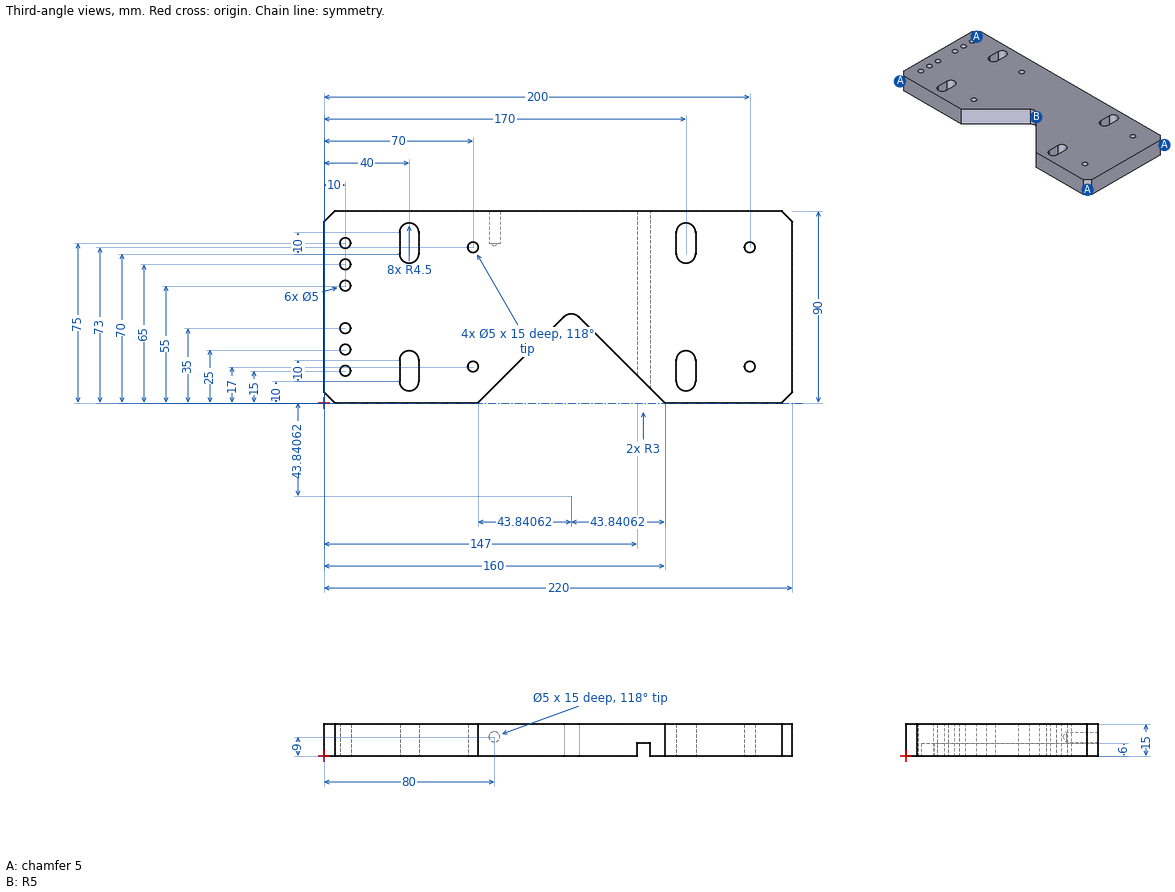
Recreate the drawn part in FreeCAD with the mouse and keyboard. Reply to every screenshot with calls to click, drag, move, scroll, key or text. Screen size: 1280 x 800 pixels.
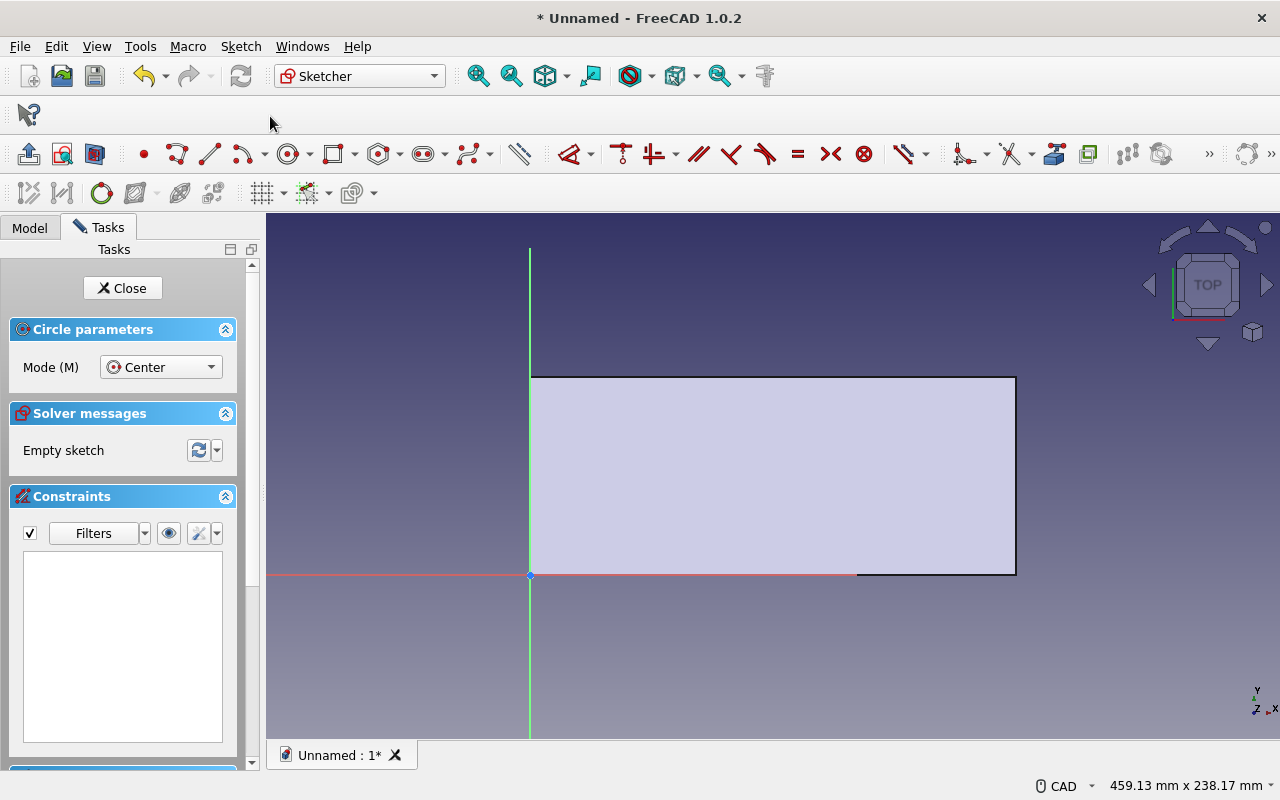
scroll(685, 414, up, 8)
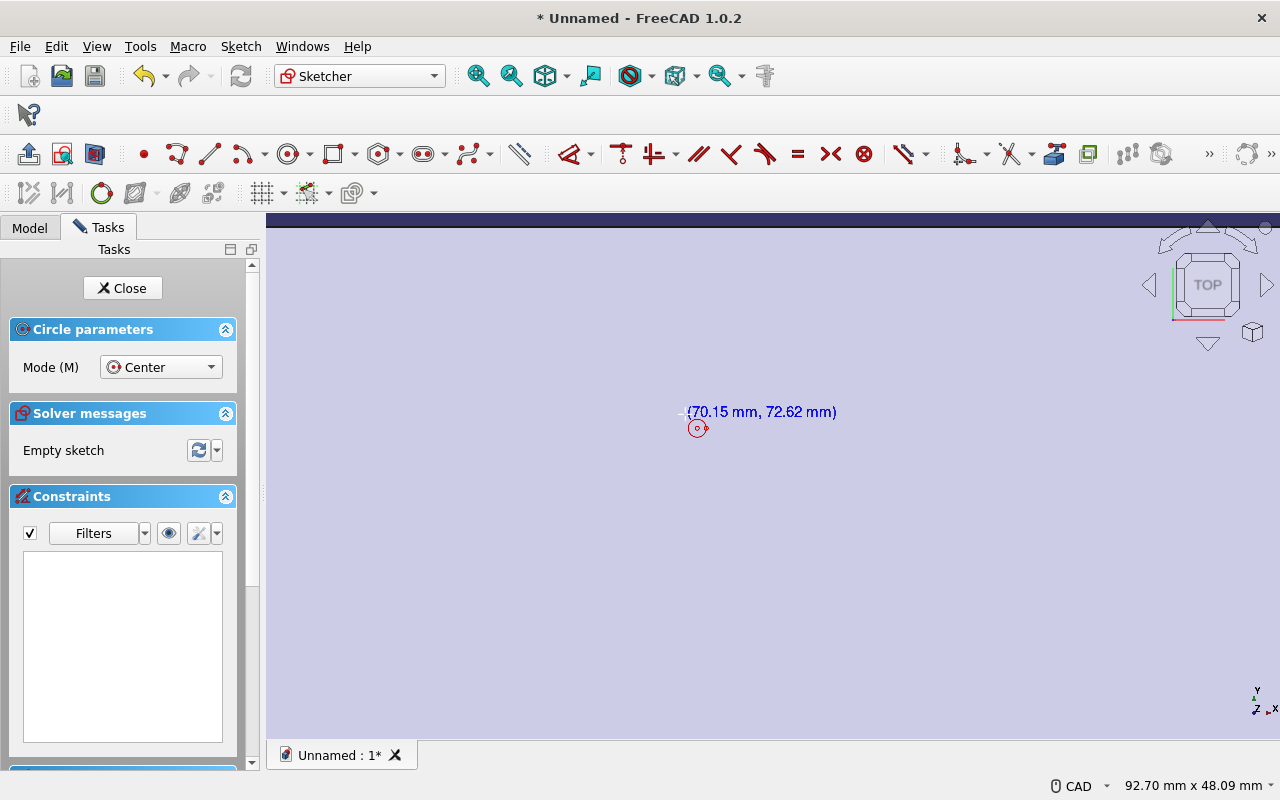
scroll(600, 370, down, 7)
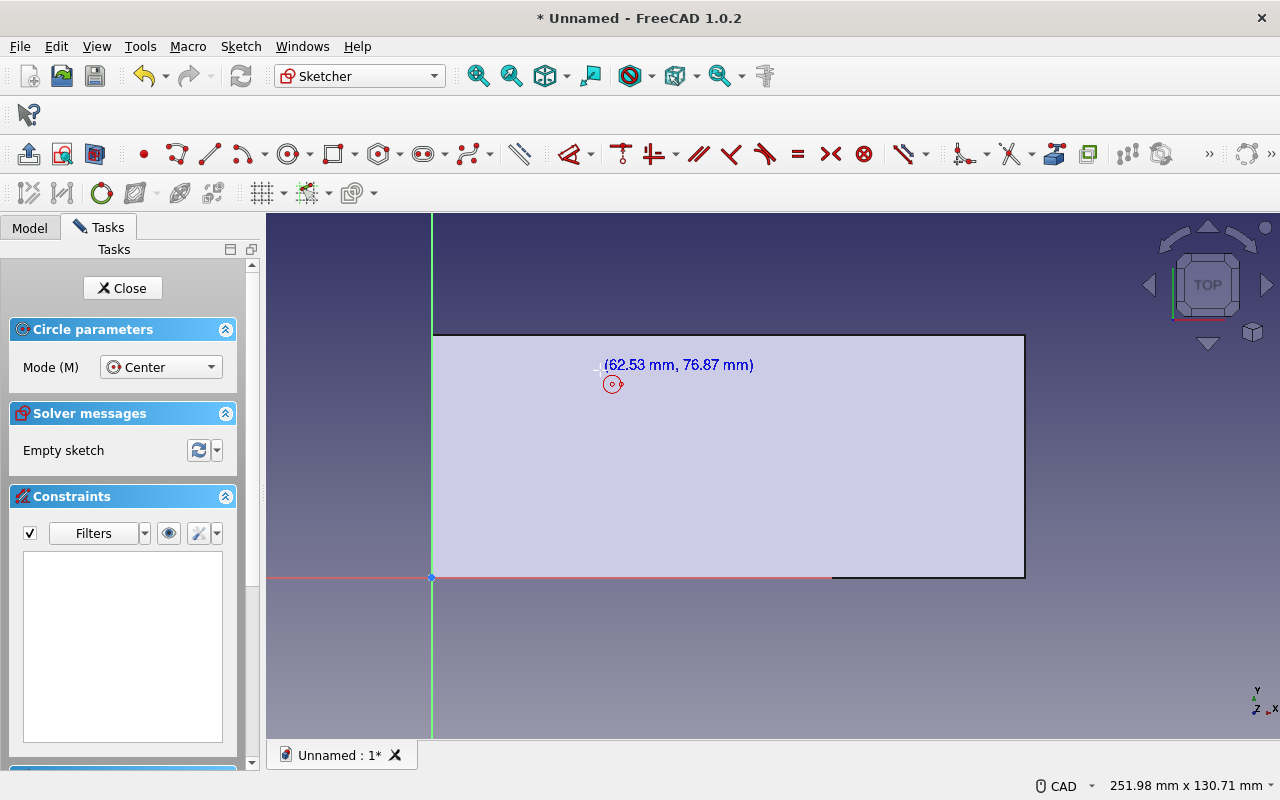
click(620, 381)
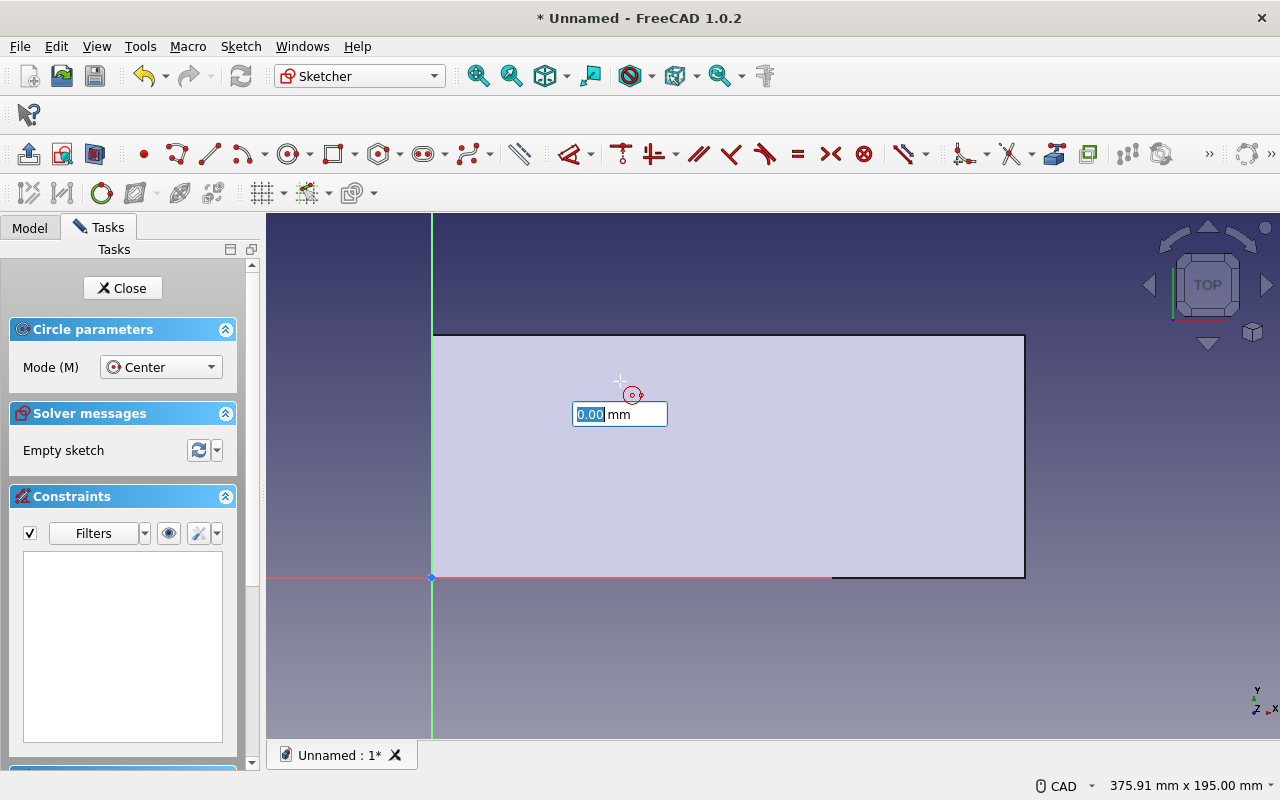
scroll(625, 376, up, 5)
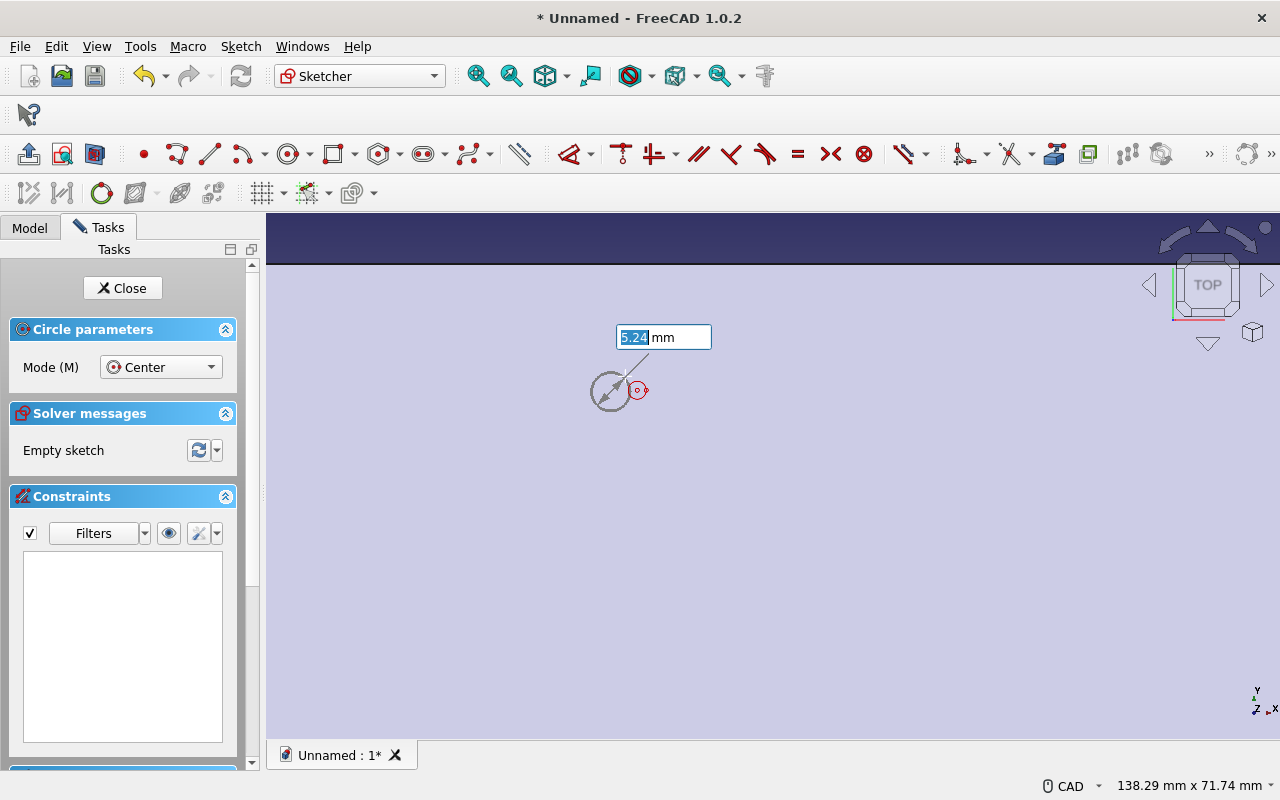
click(625, 376)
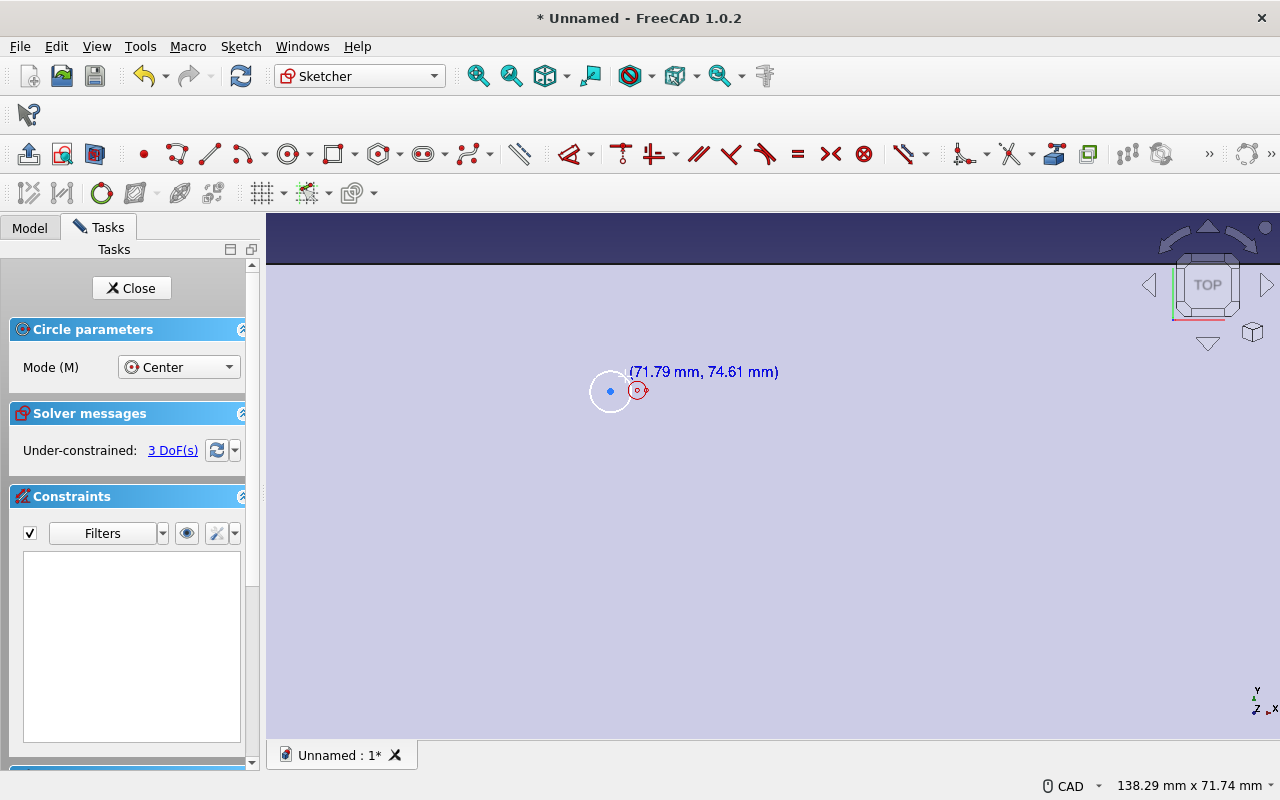
scroll(625, 376, down, 5)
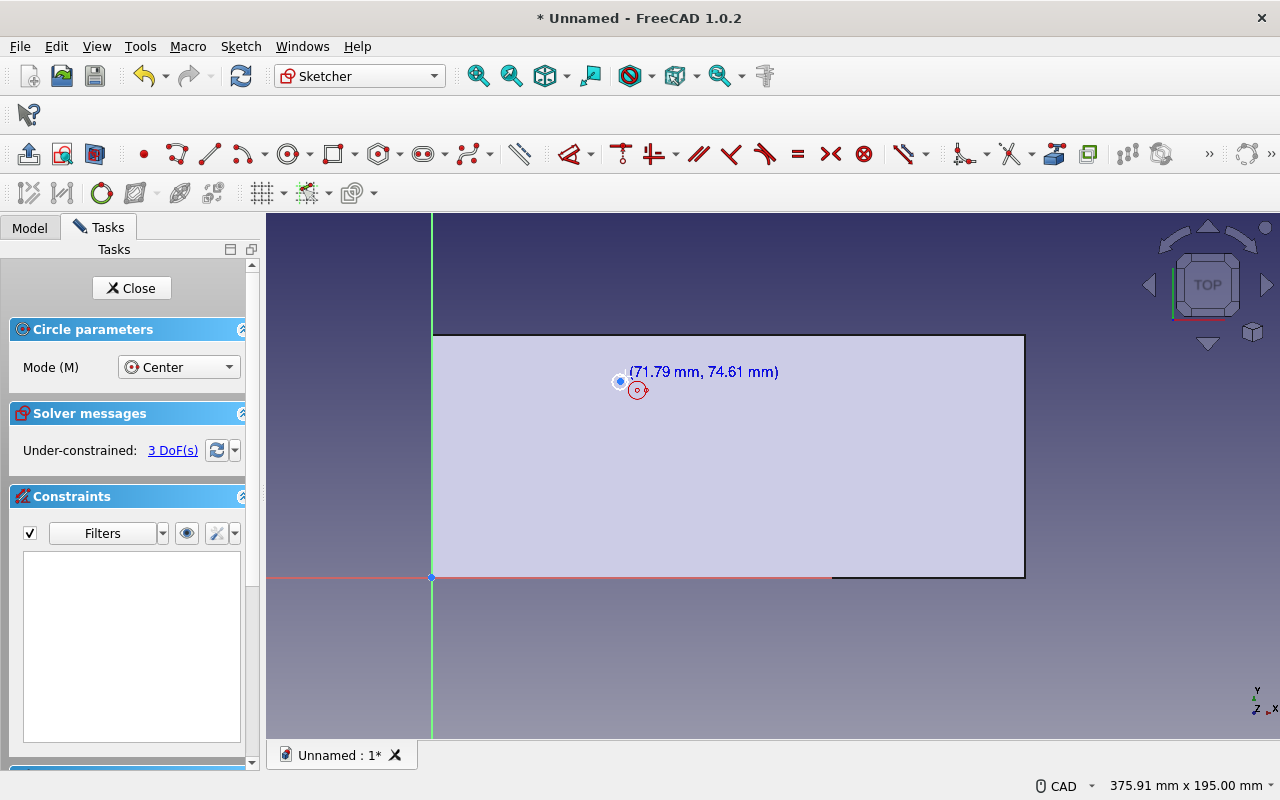
scroll(620, 532, up, 7)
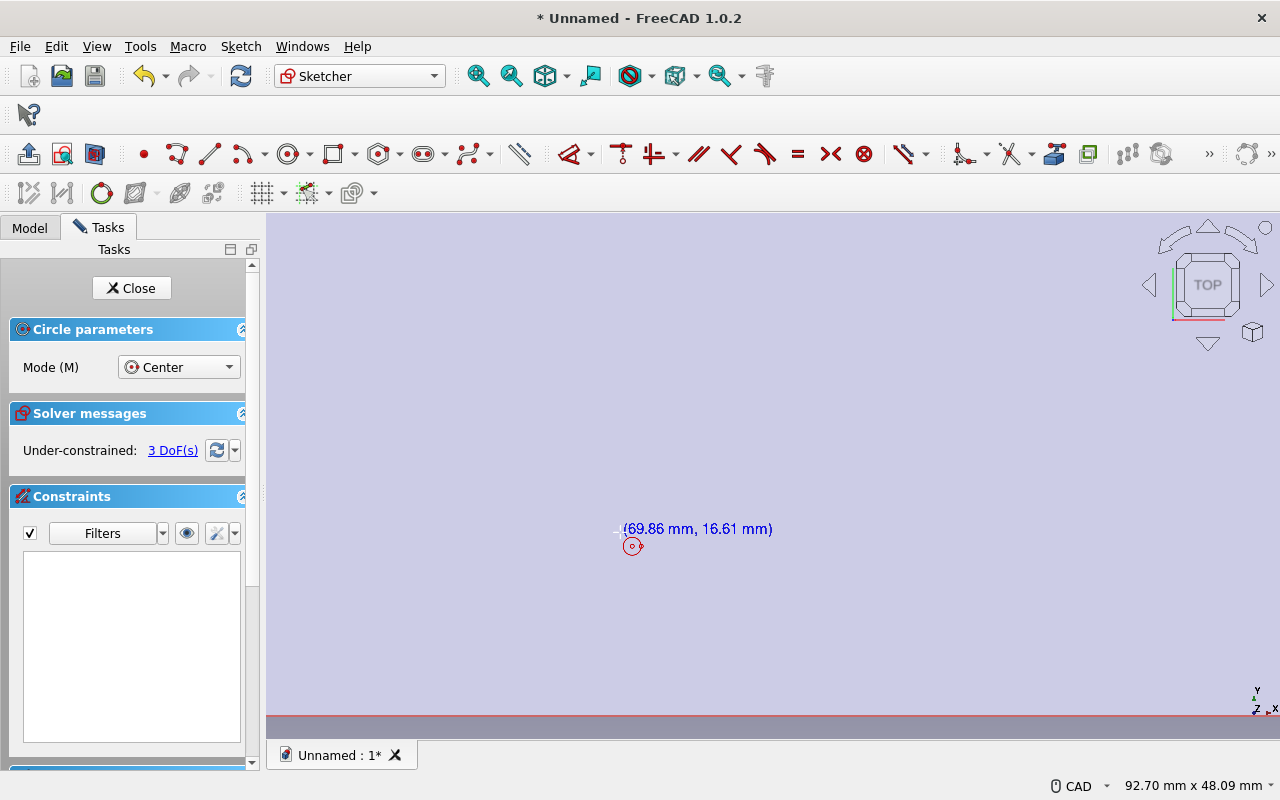
scroll(620, 533, down, 7)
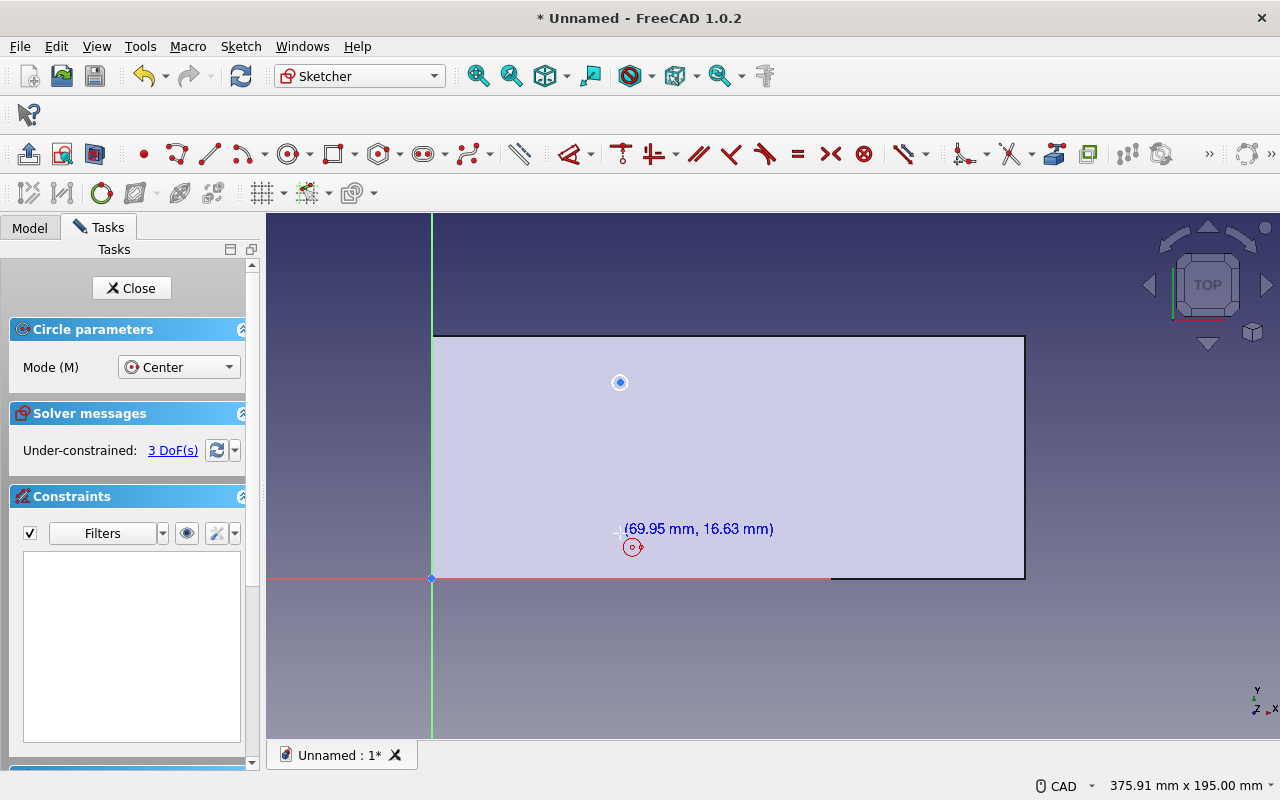
click(620, 533)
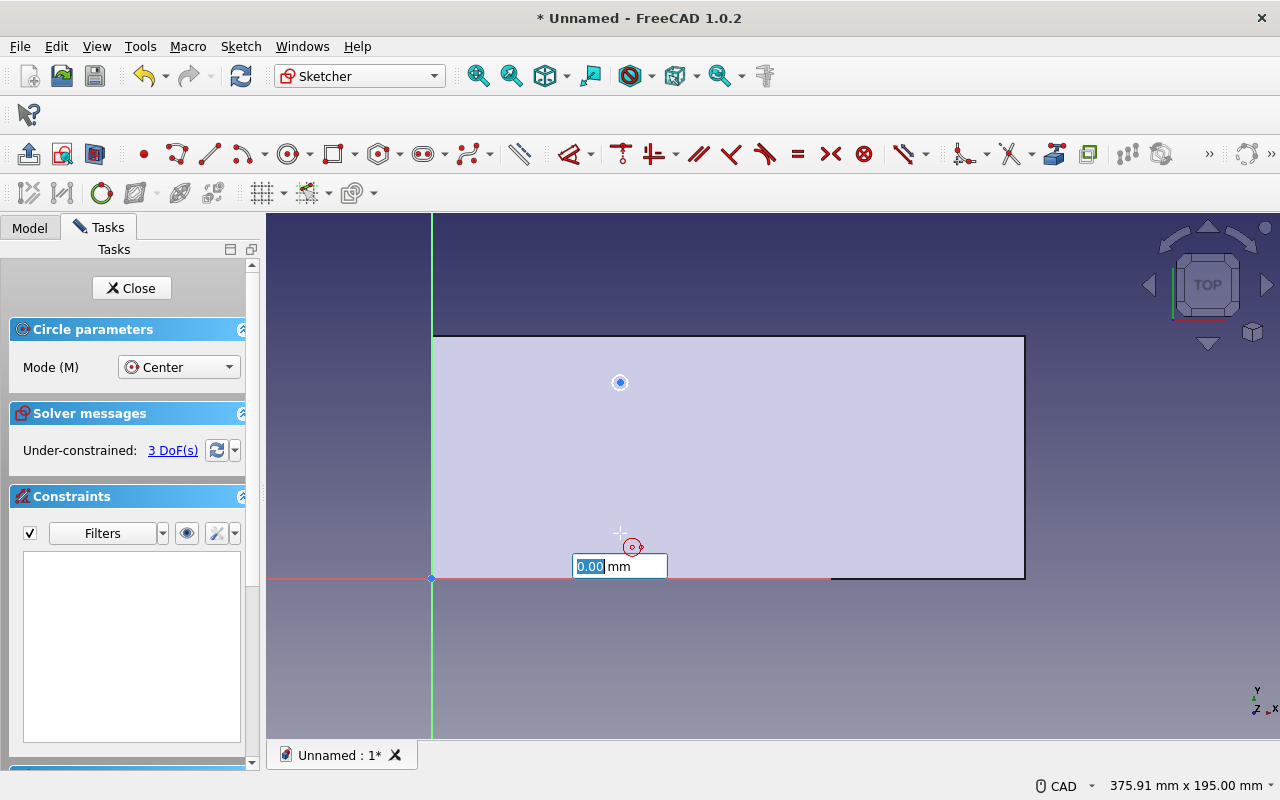
scroll(625, 528, up, 5)